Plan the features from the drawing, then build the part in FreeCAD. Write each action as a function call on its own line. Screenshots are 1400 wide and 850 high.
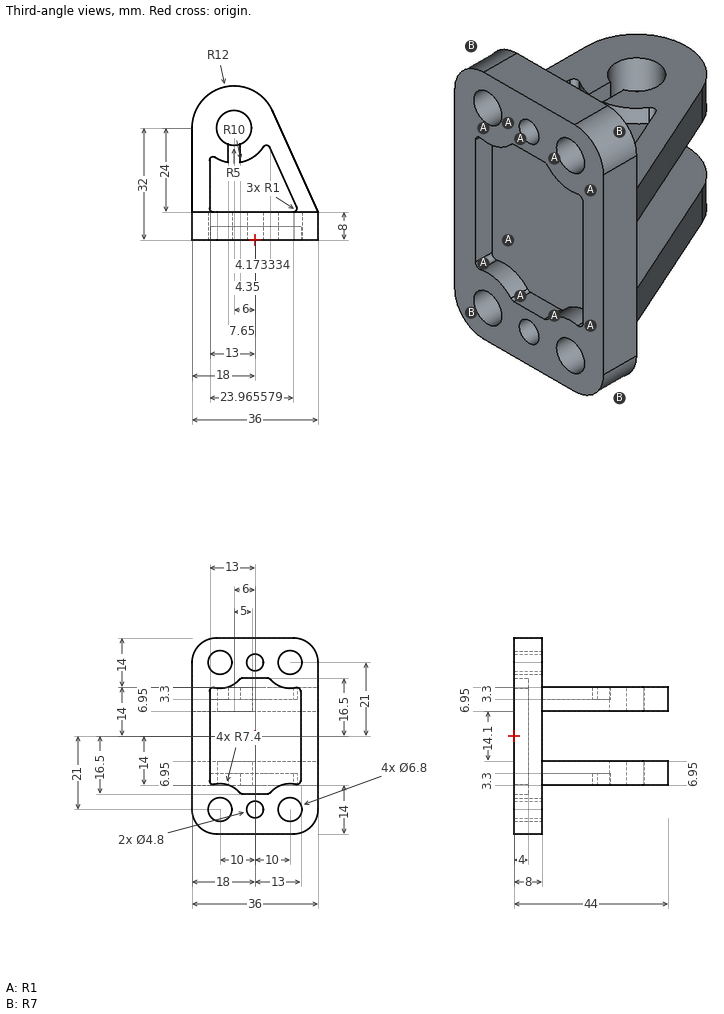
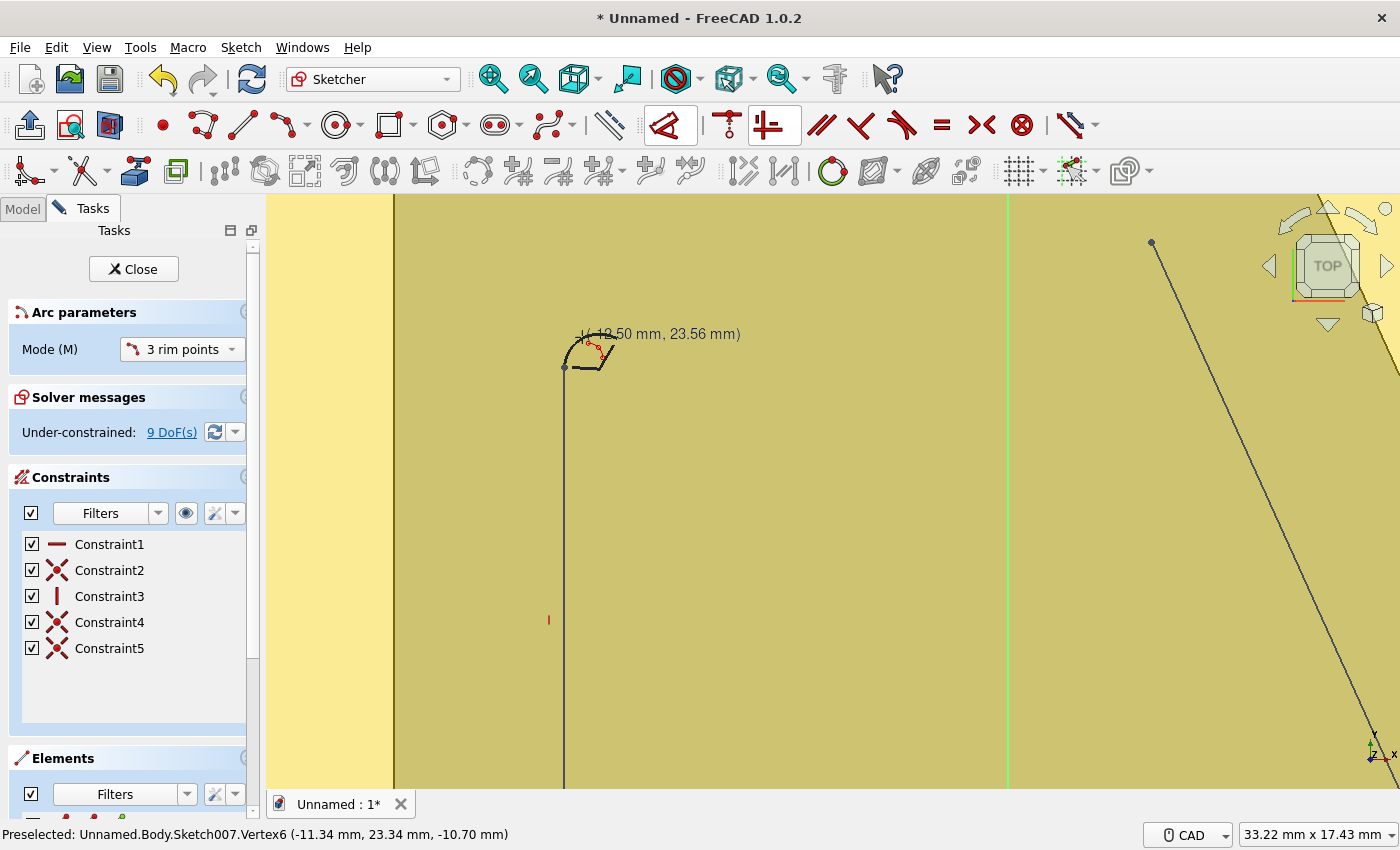
click(583, 336)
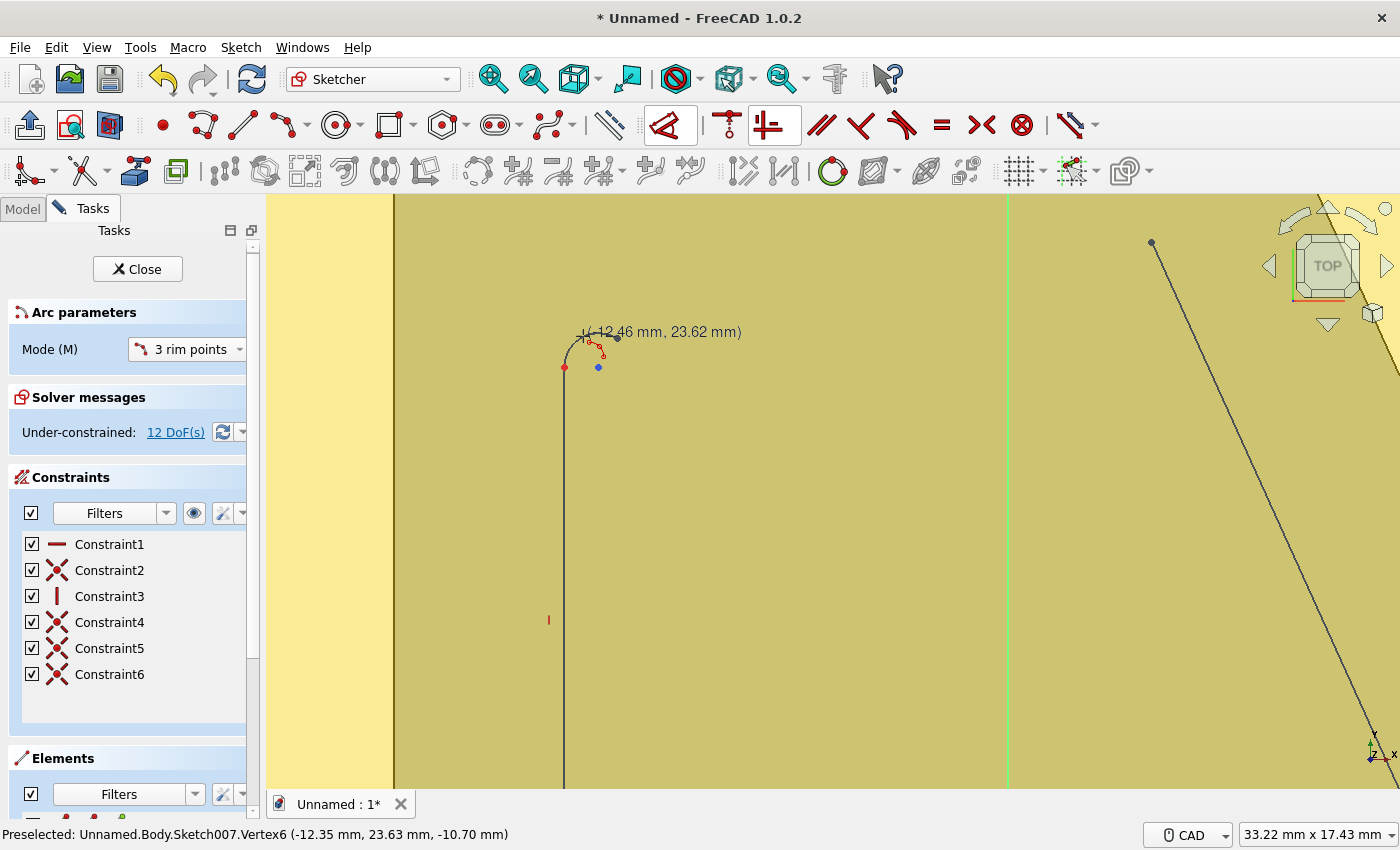
click(617, 339)
click(1091, 235)
click(875, 385)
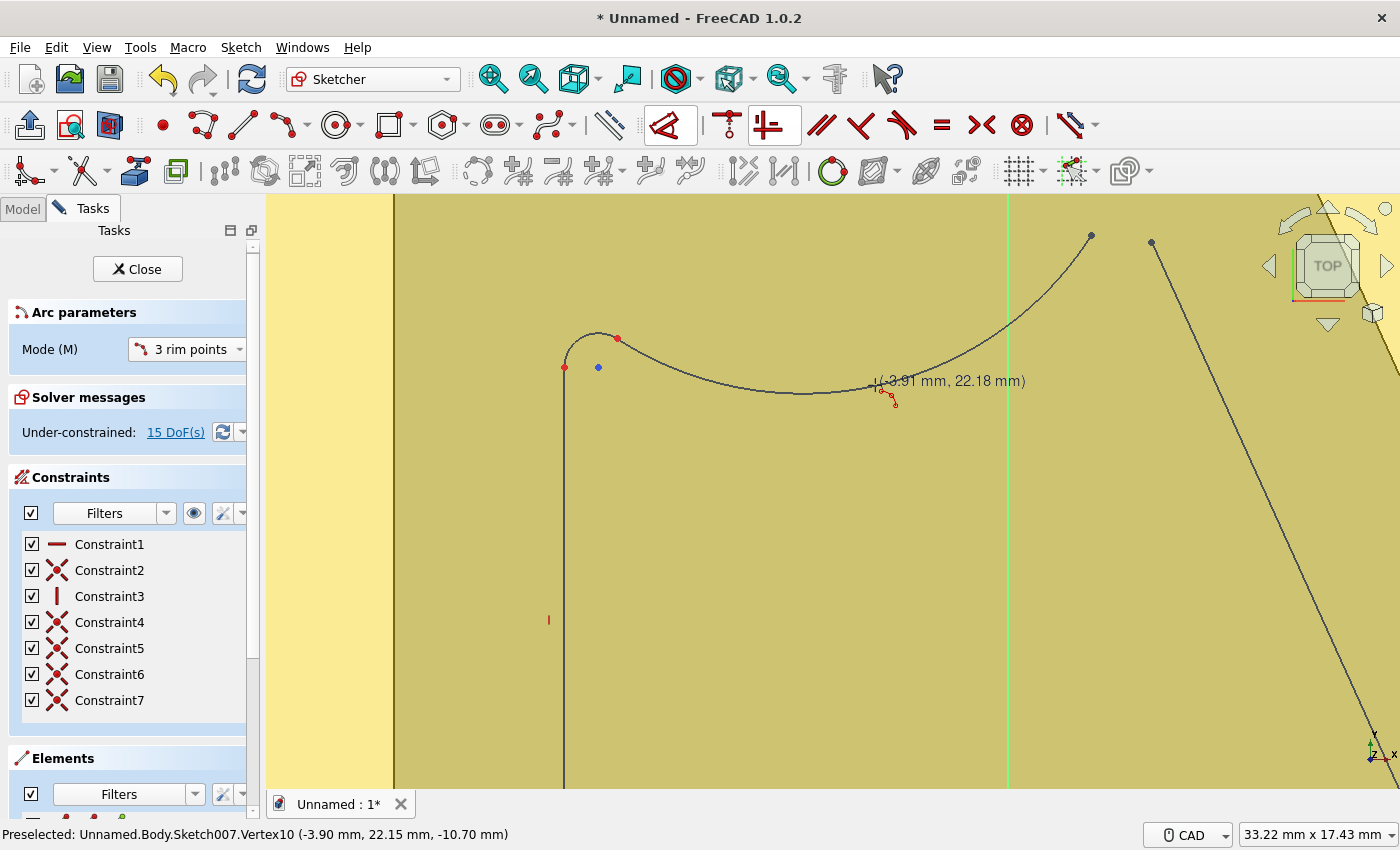
click(1091, 236)
click(1152, 242)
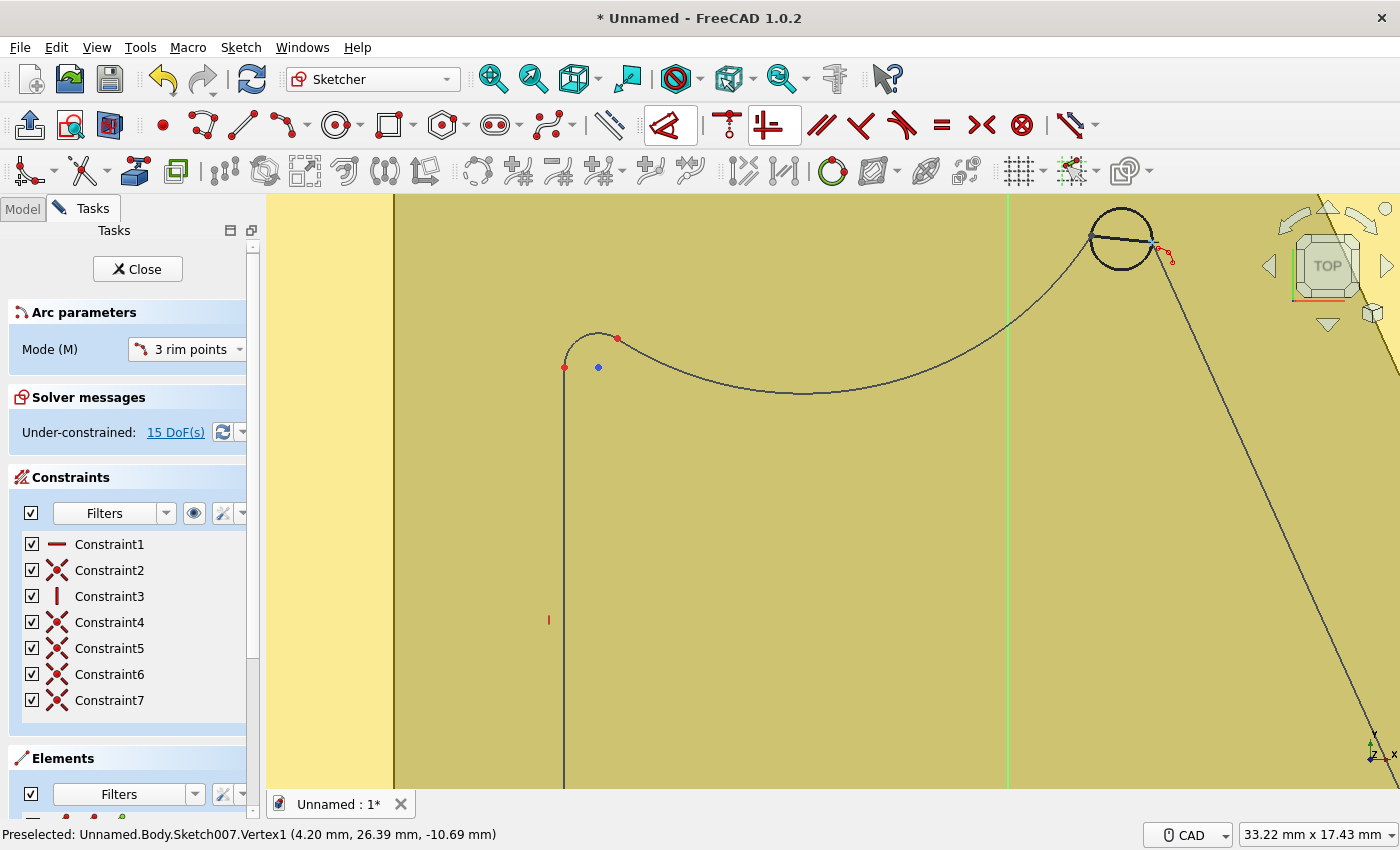
scroll(581, 337, down, 4)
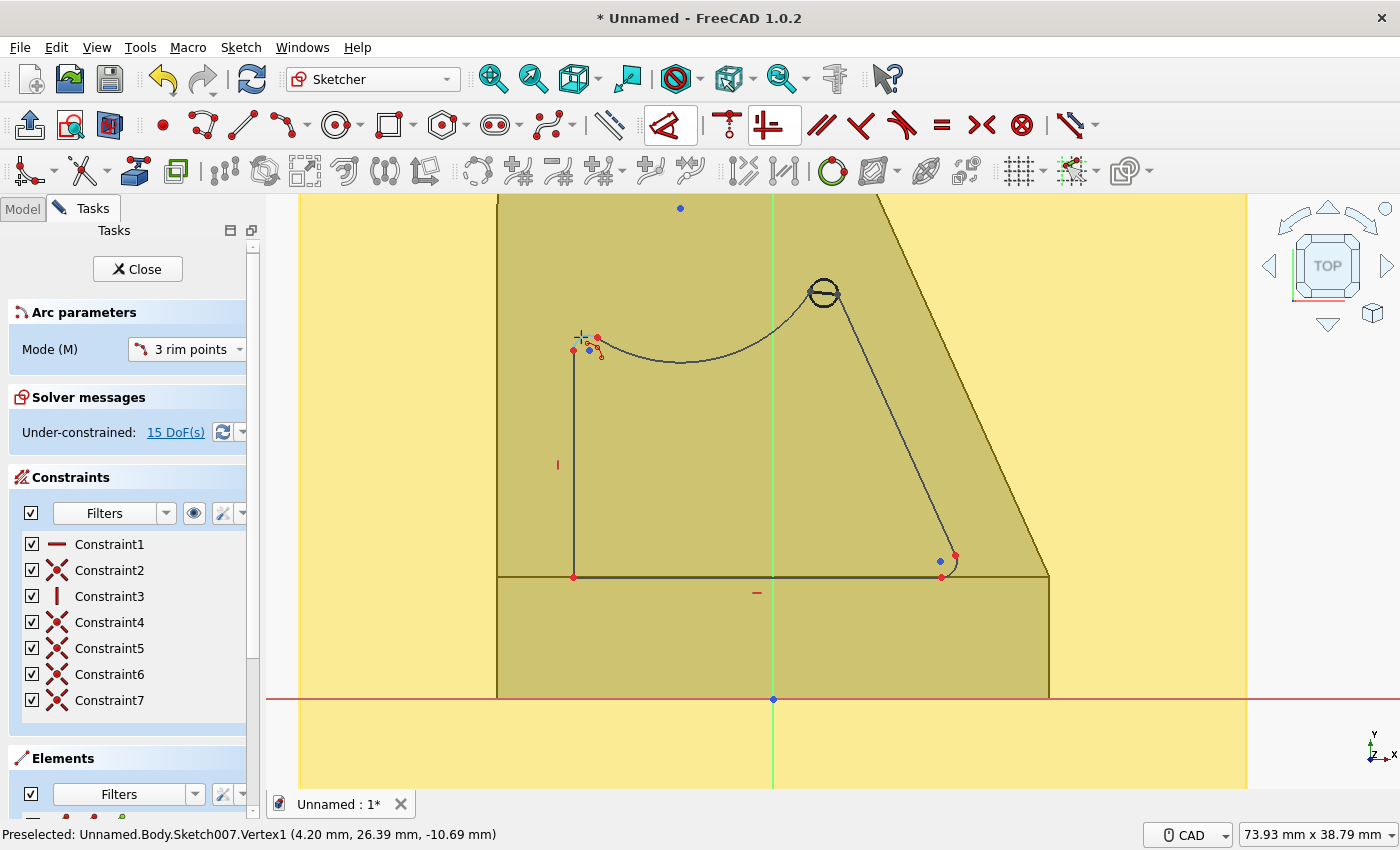
scroll(824, 284, up, 4)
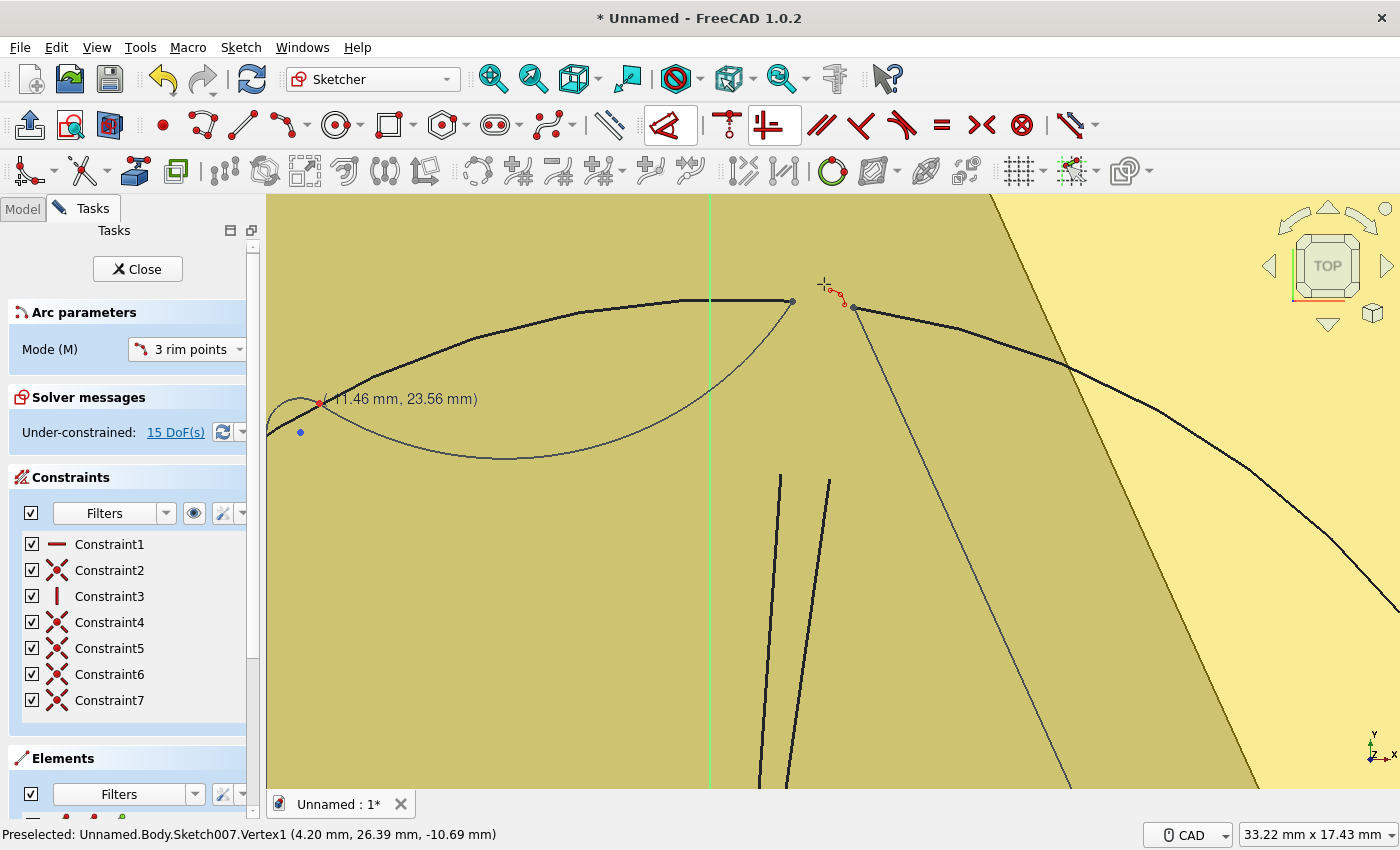
click(824, 285)
key(Escape)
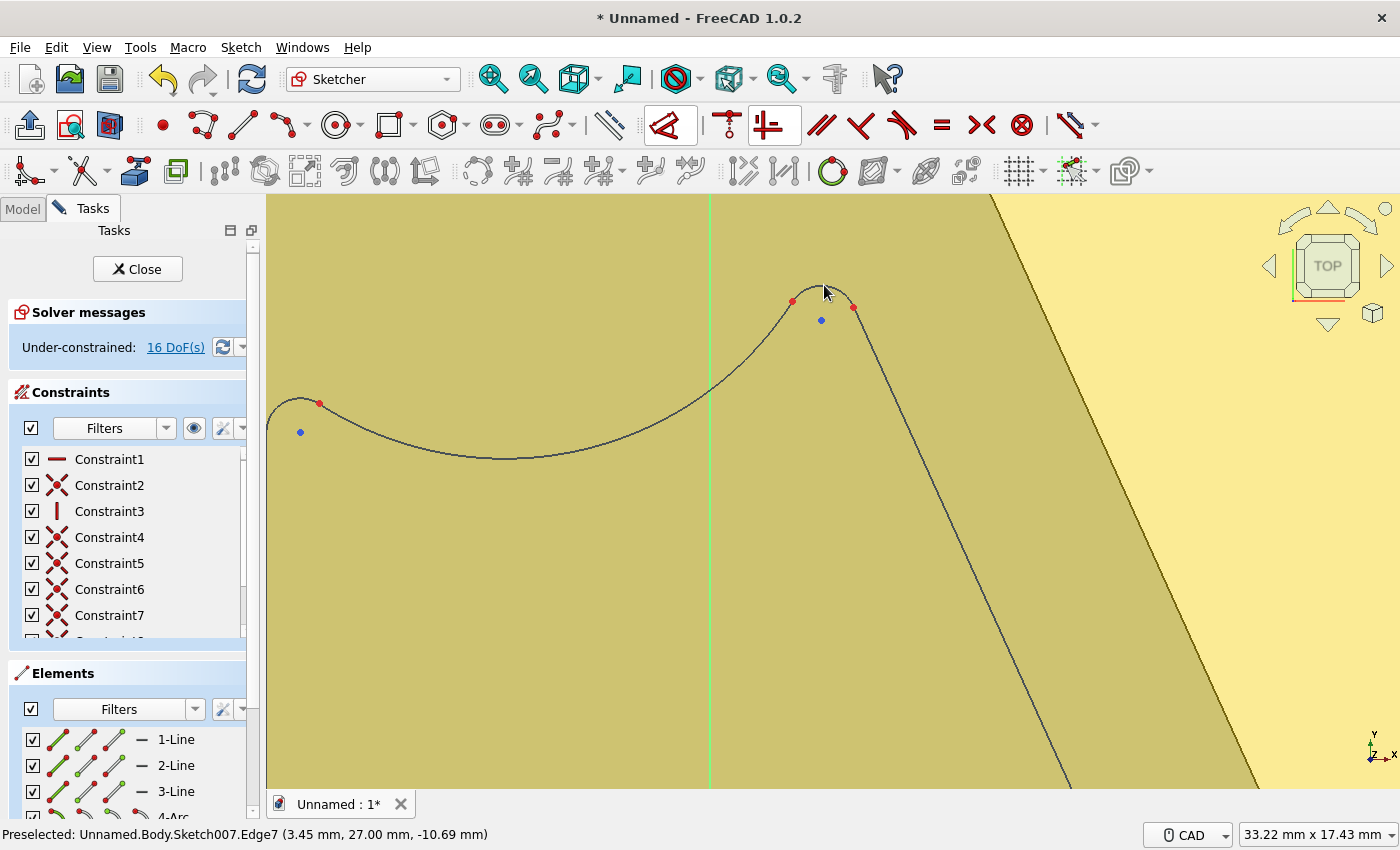
click(933, 482)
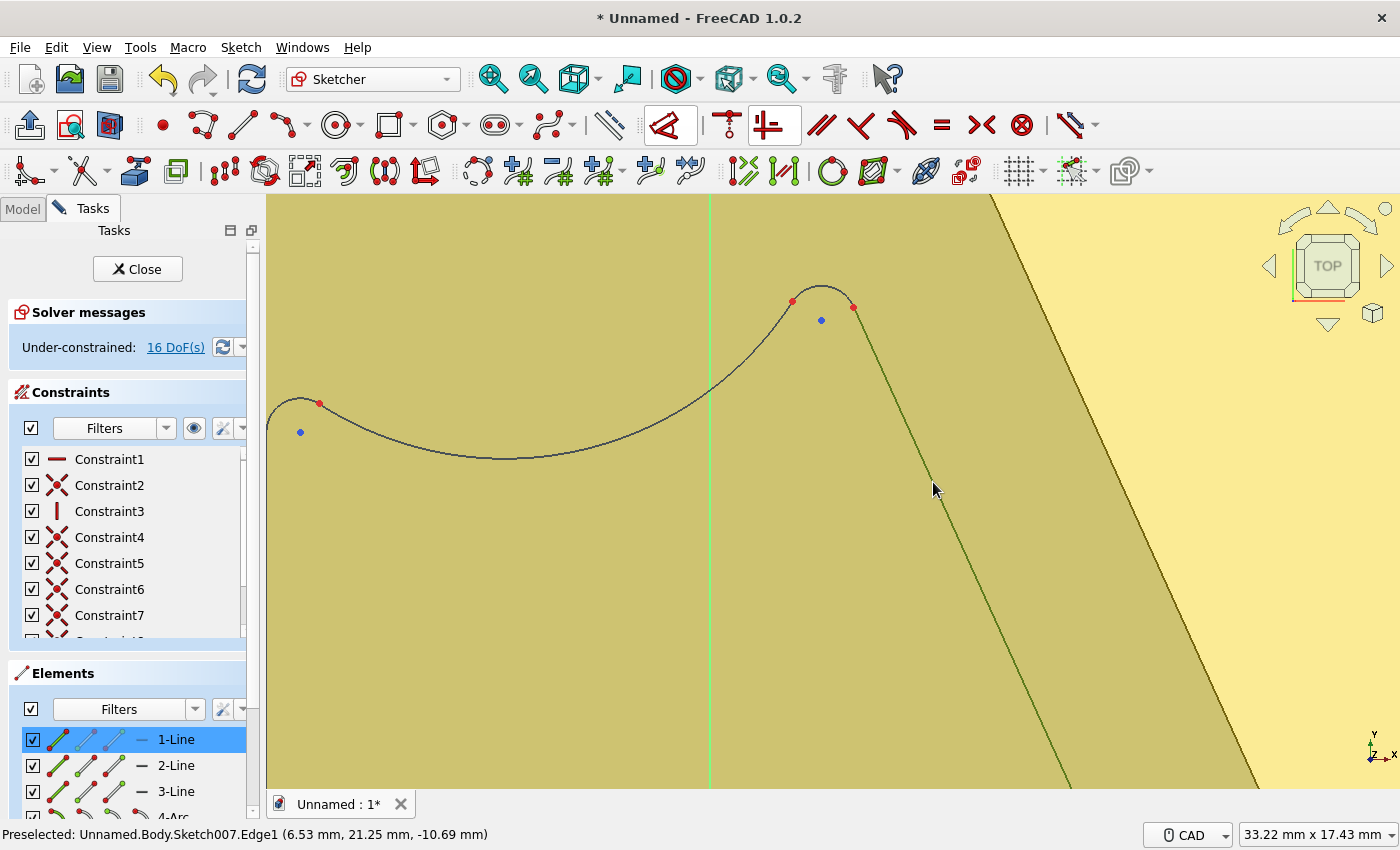
scroll(824, 283, down, 4)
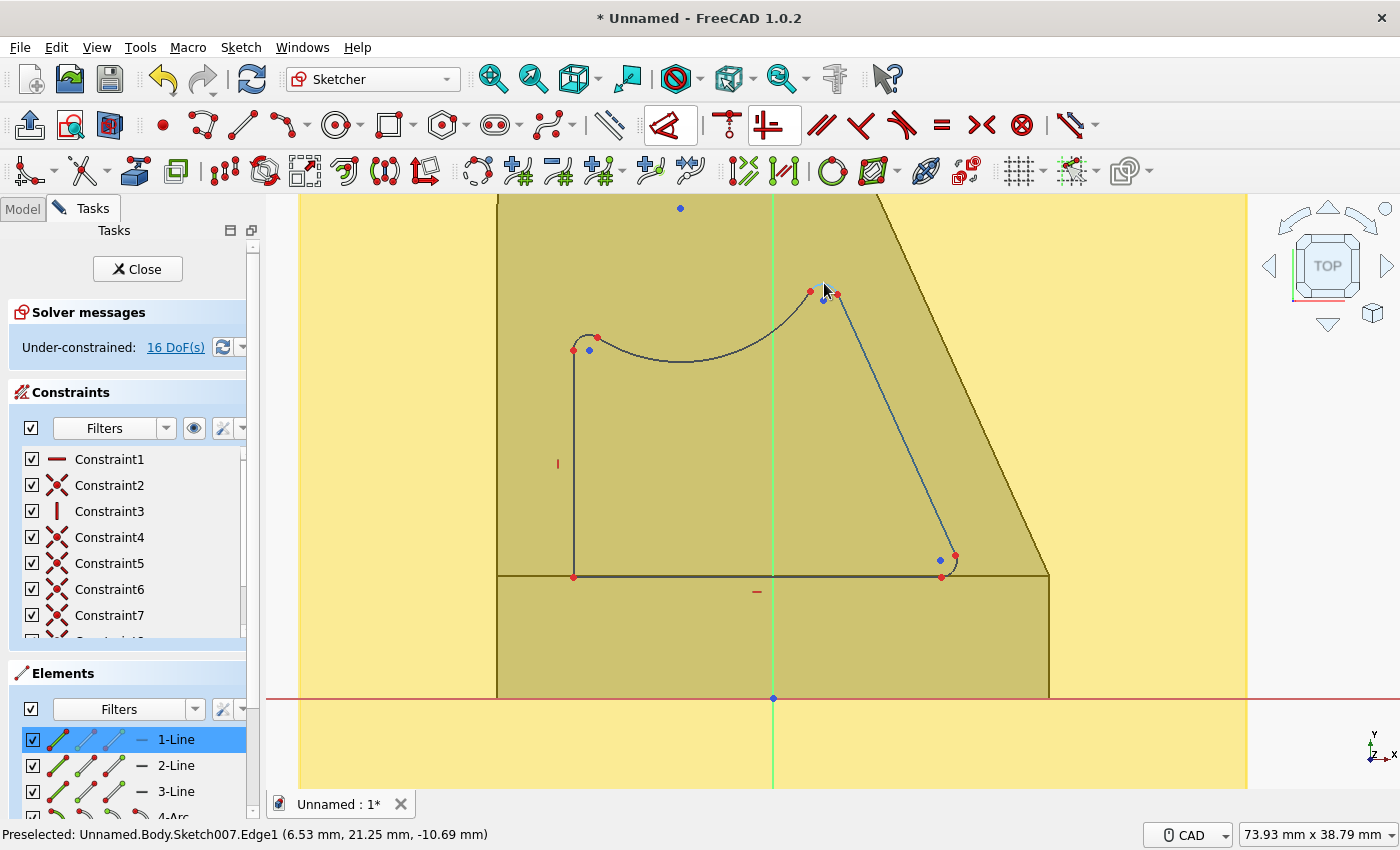
scroll(950, 574, up, 3)